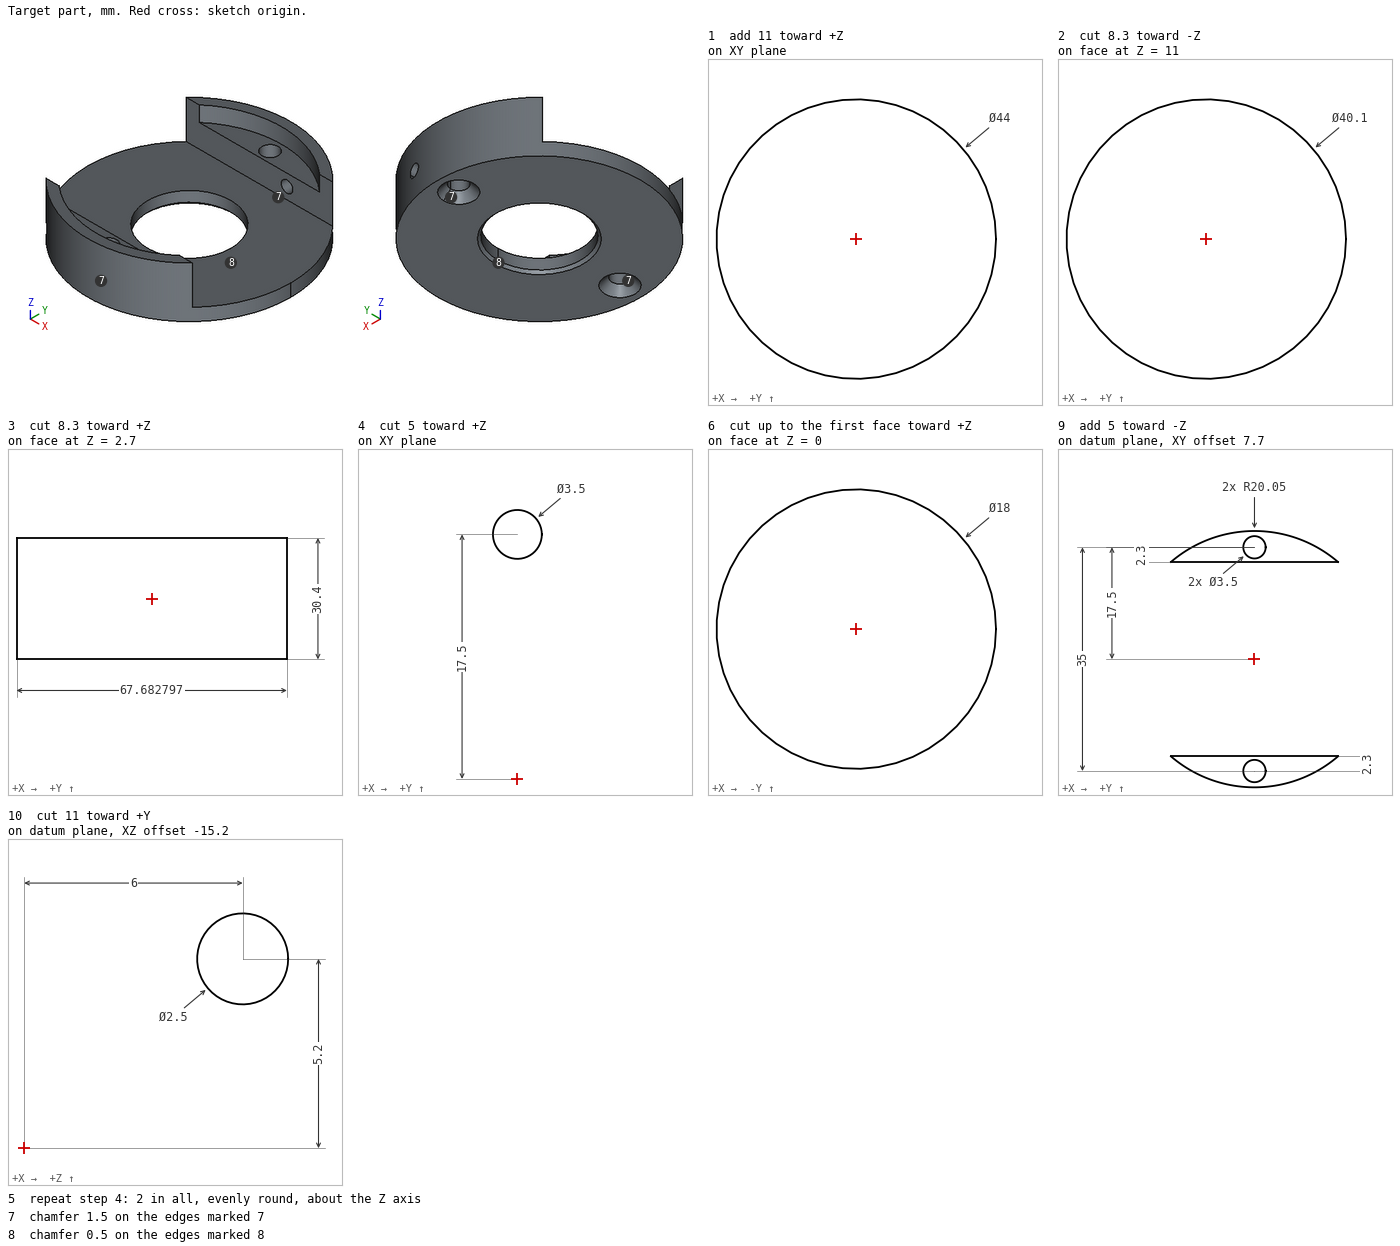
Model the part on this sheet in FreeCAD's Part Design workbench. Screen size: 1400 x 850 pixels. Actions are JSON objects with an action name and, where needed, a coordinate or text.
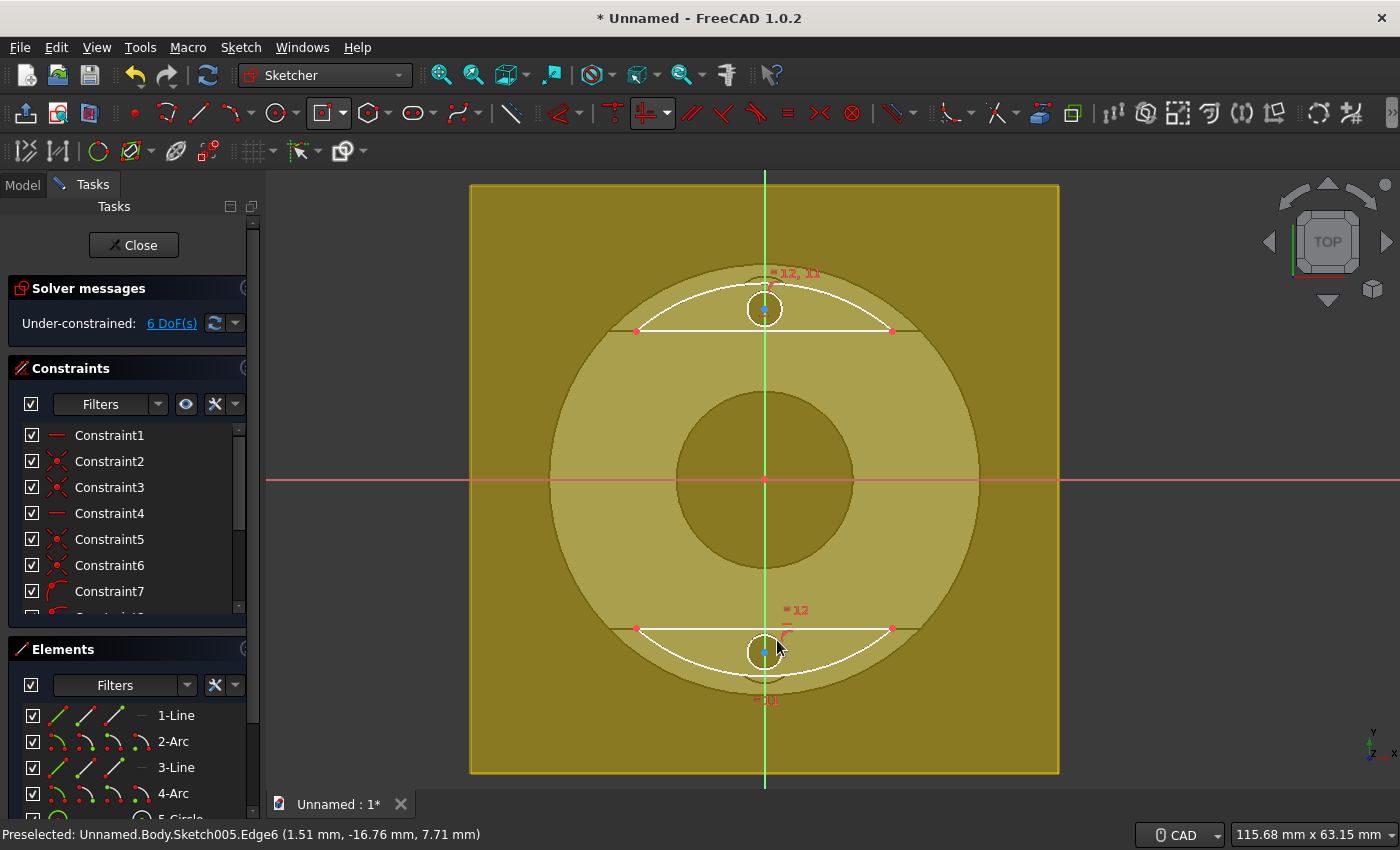
{"action": "left_click", "coordinate": [558, 114]}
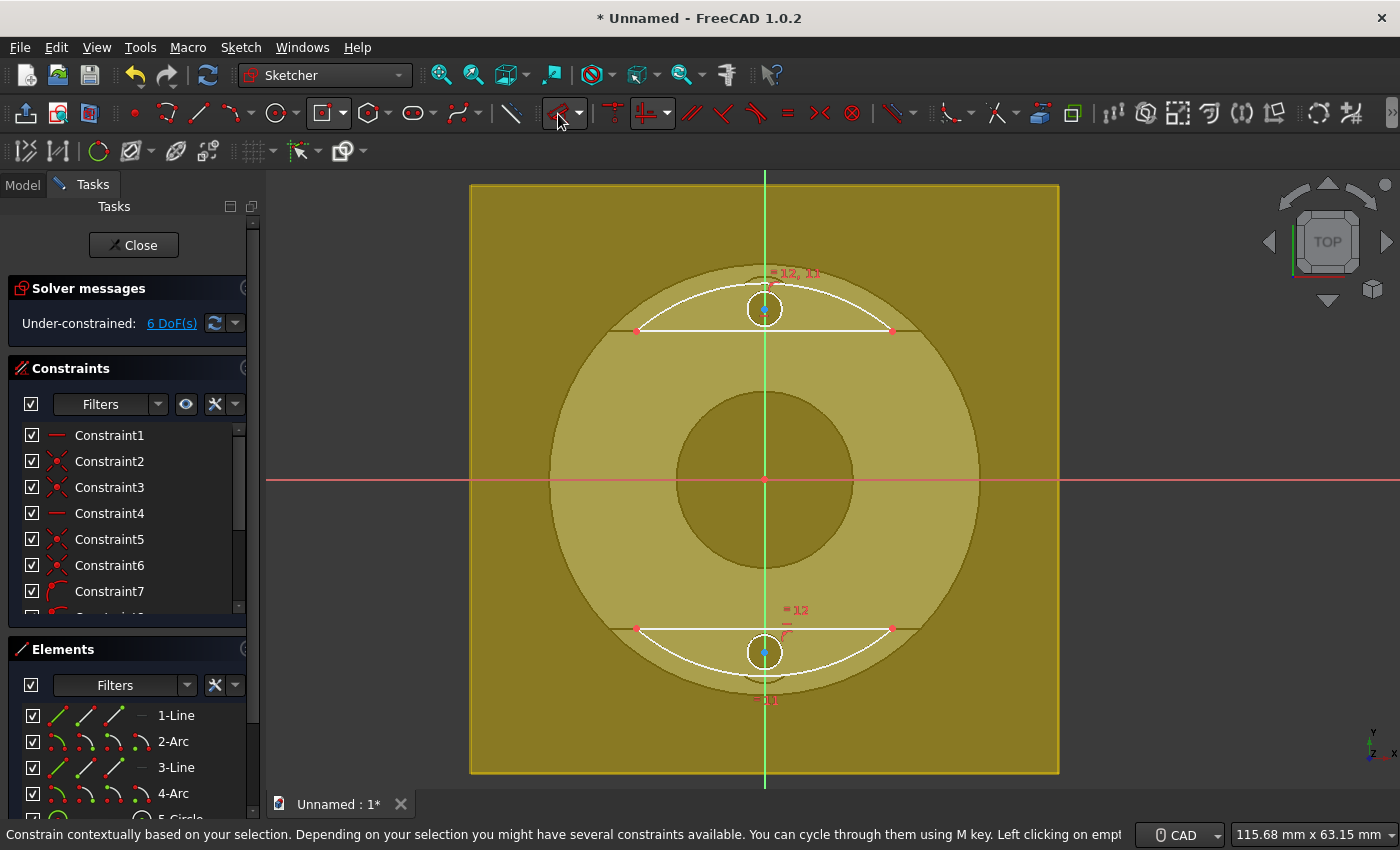
{"action": "left_click", "coordinate": [820, 291]}
{"action": "left_click", "coordinate": [829, 260]}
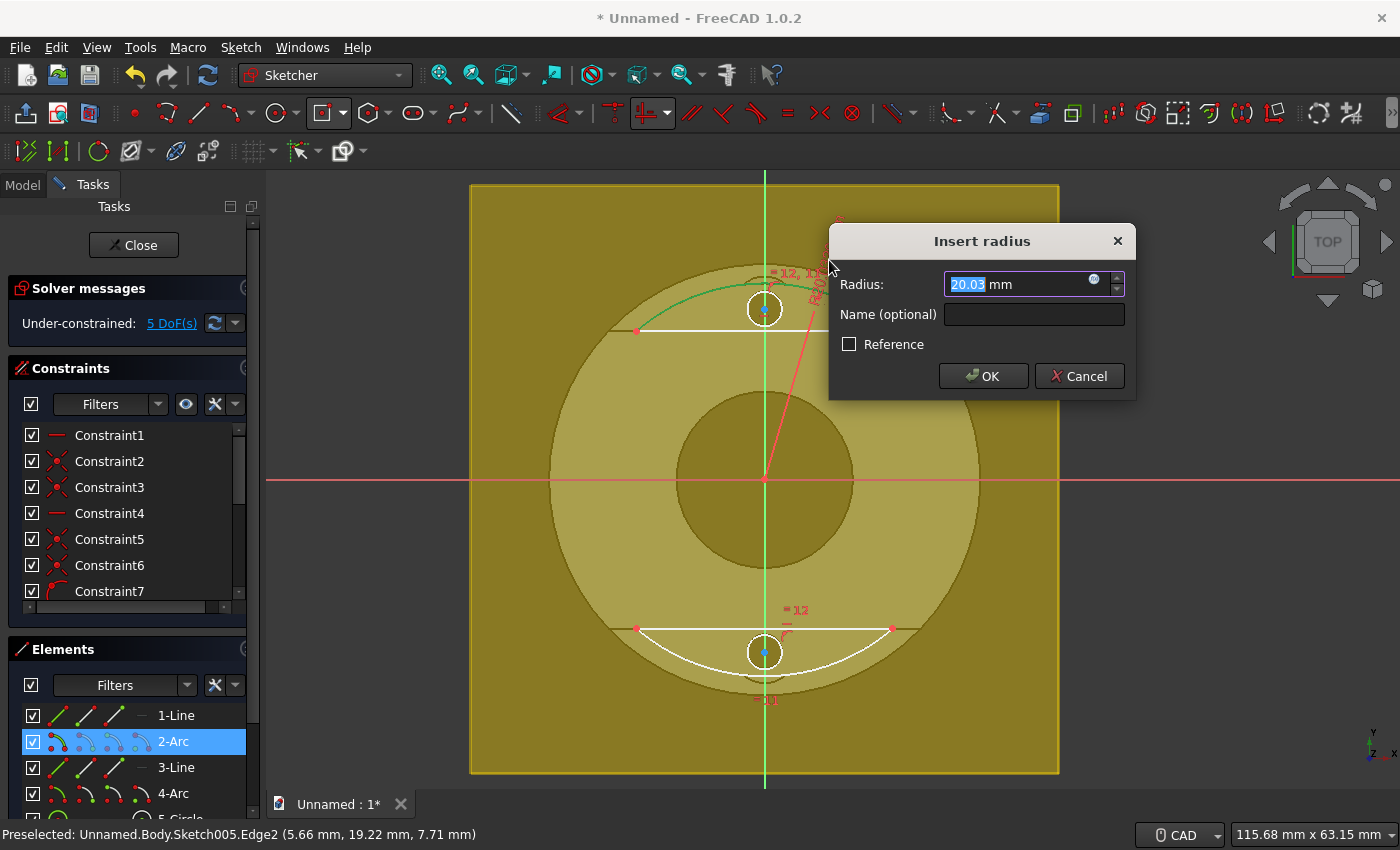
{"action": "type", "text": "20.05"}
{"action": "key", "text": "Return"}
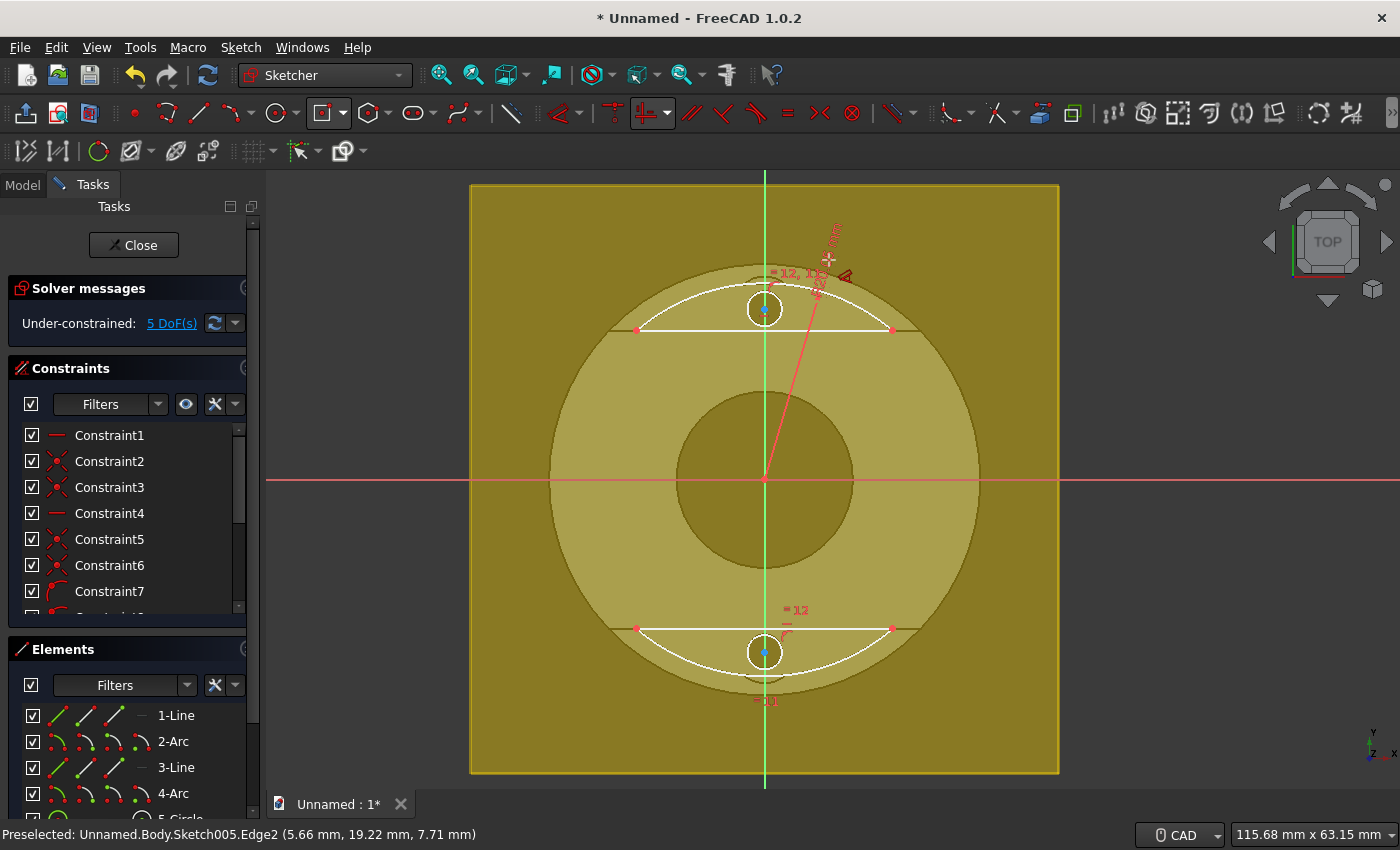
{"action": "left_click", "coordinate": [777, 297]}
{"action": "left_click", "coordinate": [799, 344]}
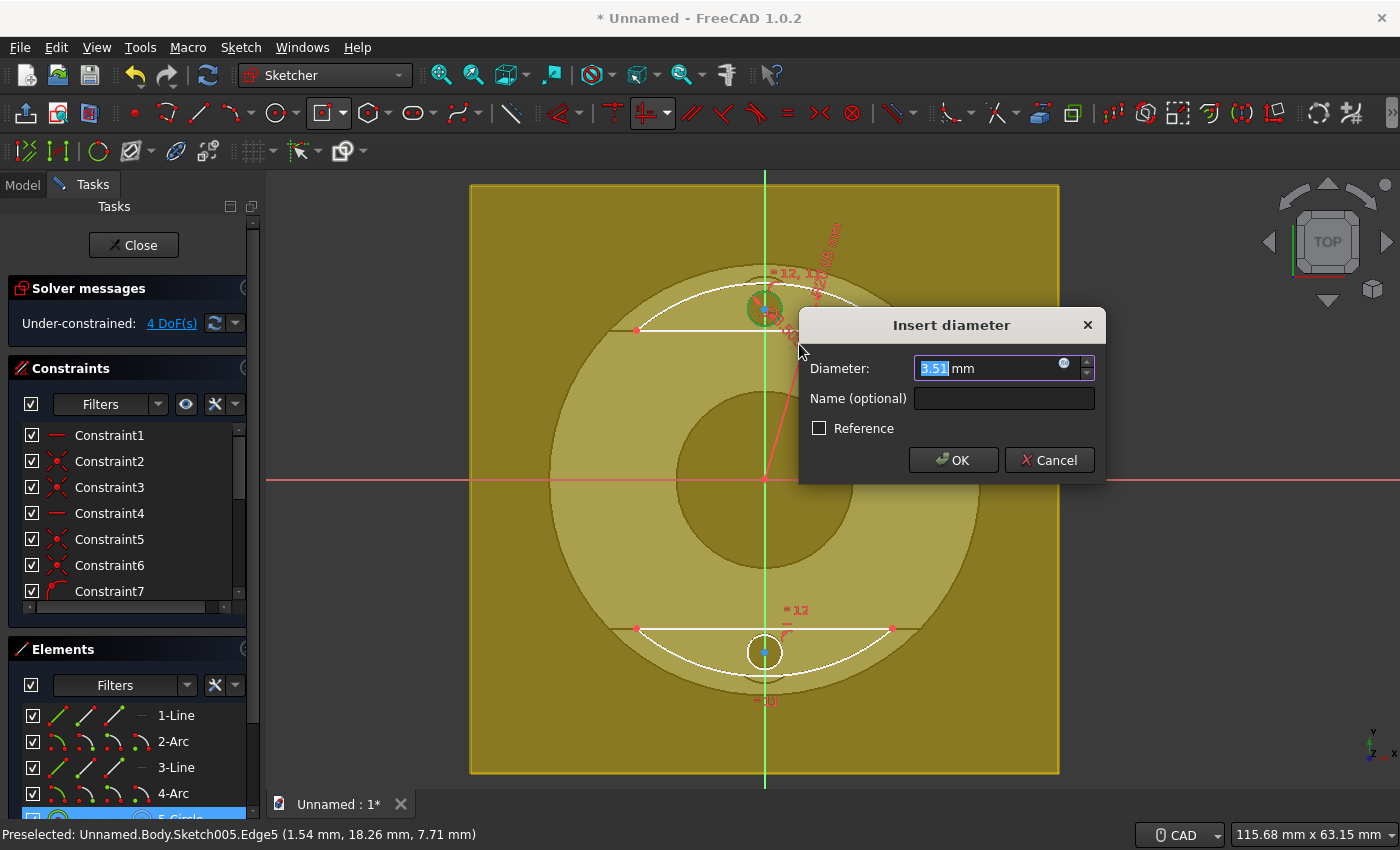
{"action": "type", "text": "3.5"}
{"action": "key", "text": "Return"}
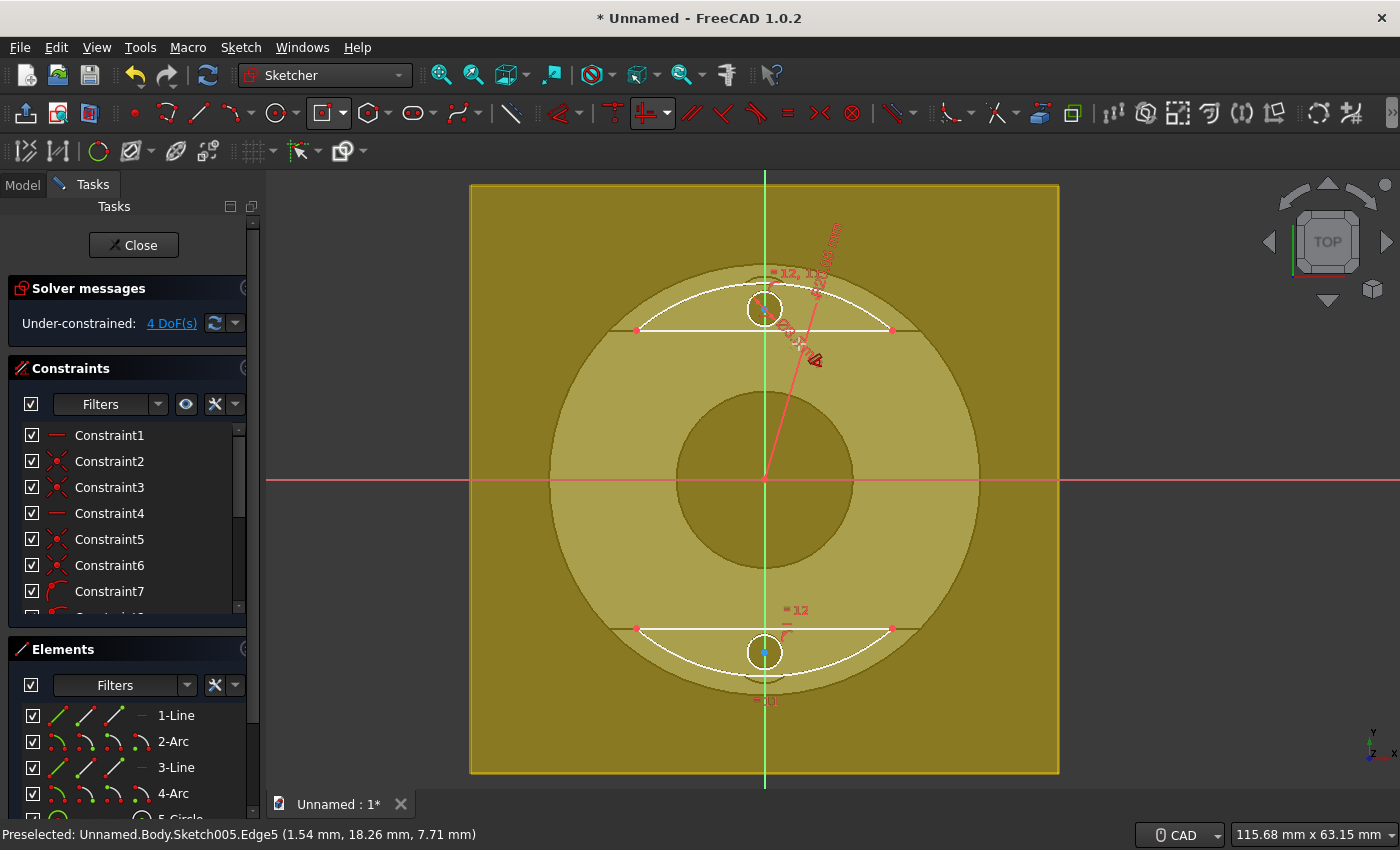
{"action": "left_click", "coordinate": [765, 309]}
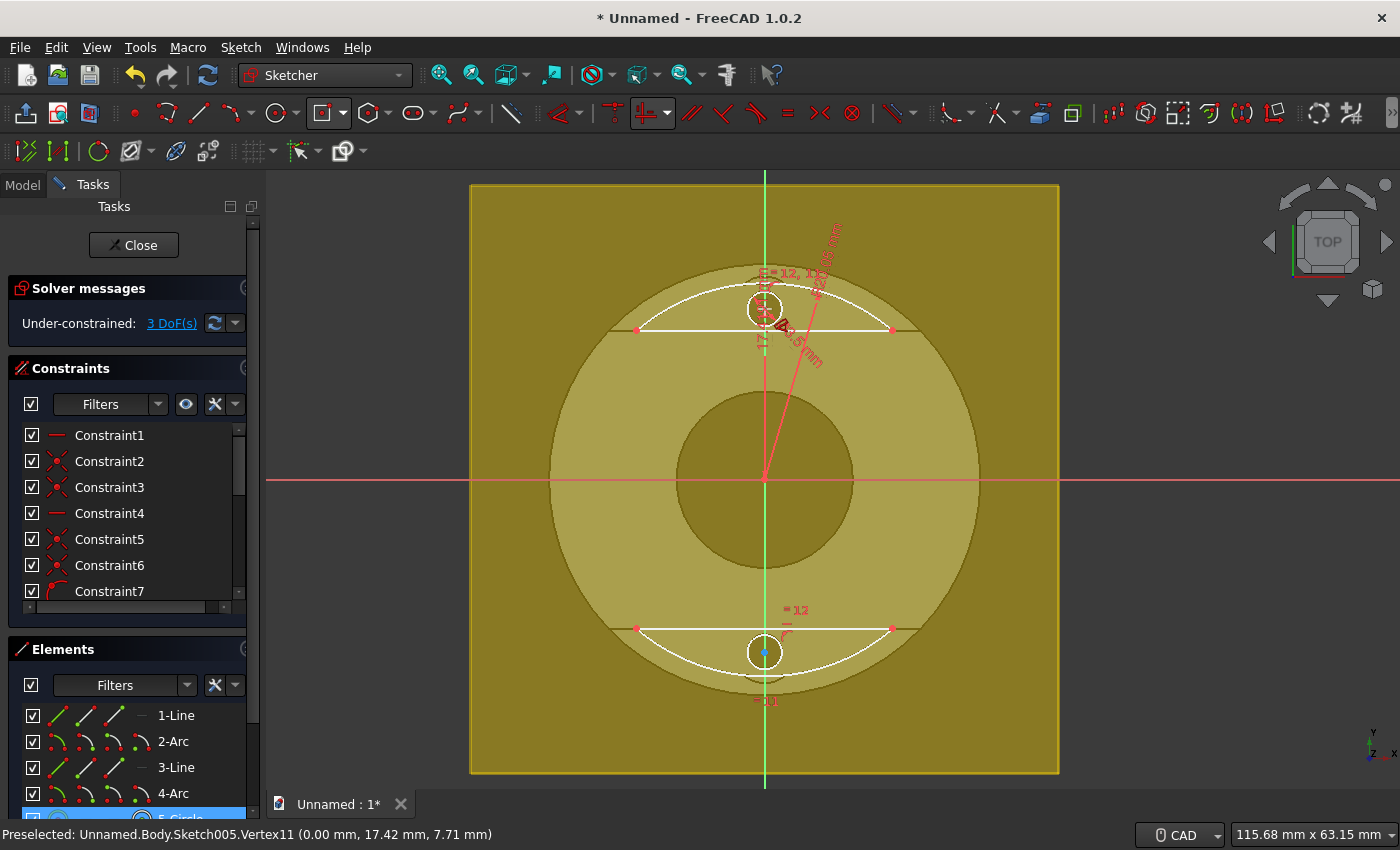
{"action": "left_click", "coordinate": [765, 652]}
{"action": "left_click", "coordinate": [799, 402]}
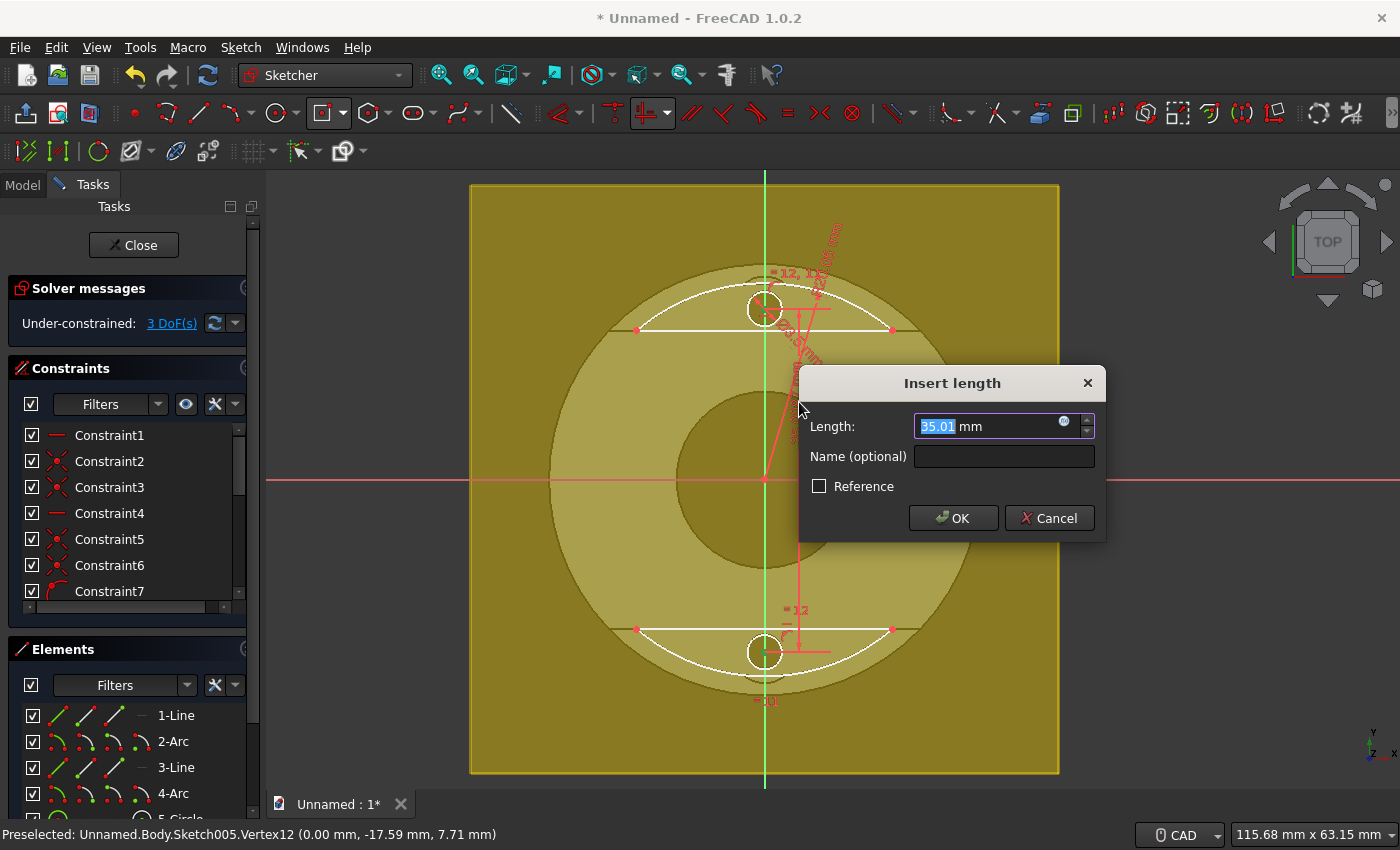
{"action": "type", "text": "35"}
{"action": "key", "text": "Return"}